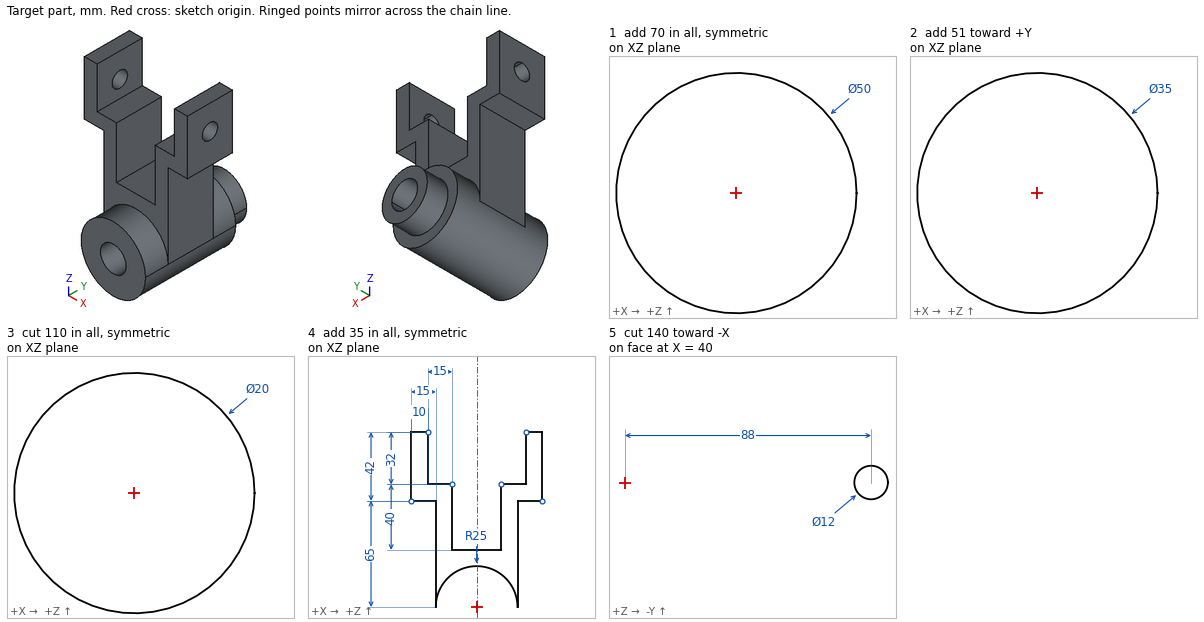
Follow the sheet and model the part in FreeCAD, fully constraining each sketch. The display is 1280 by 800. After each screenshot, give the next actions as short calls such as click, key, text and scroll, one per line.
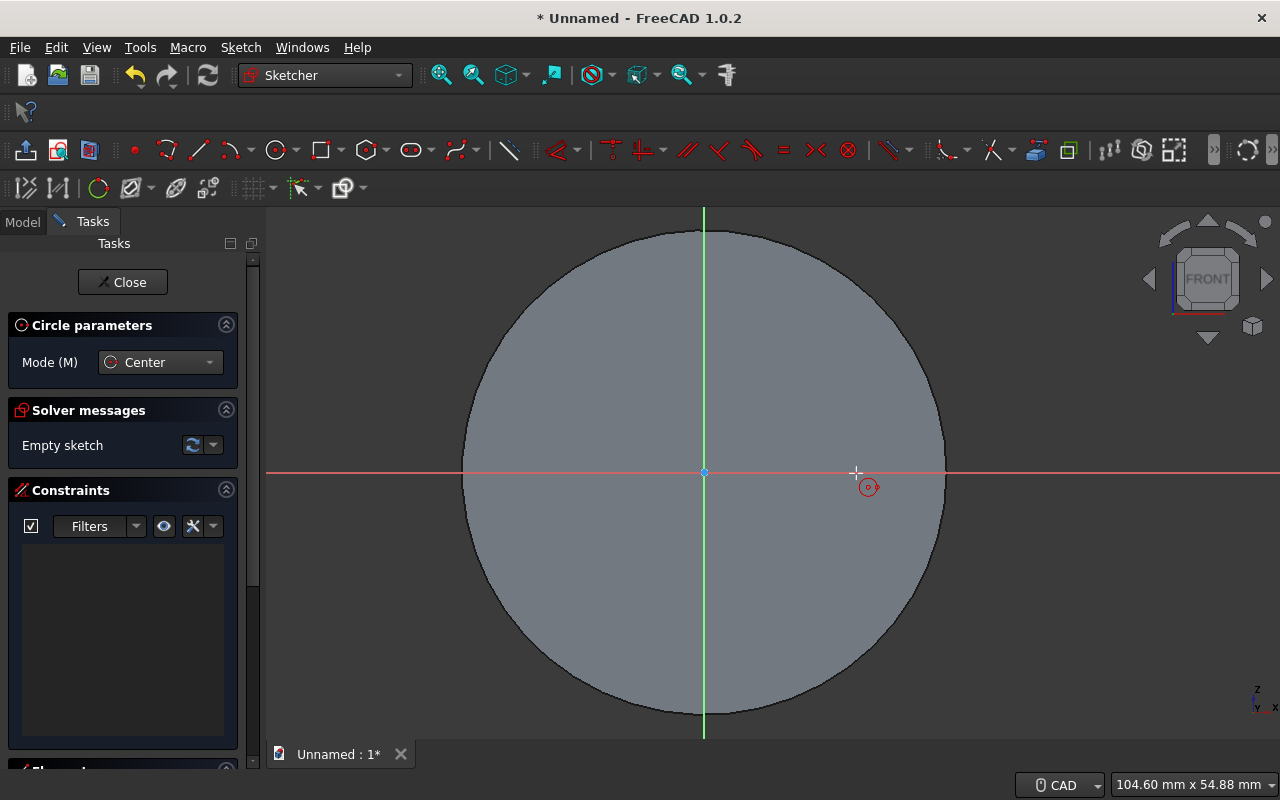
click(704, 473)
click(824, 353)
key(Escape)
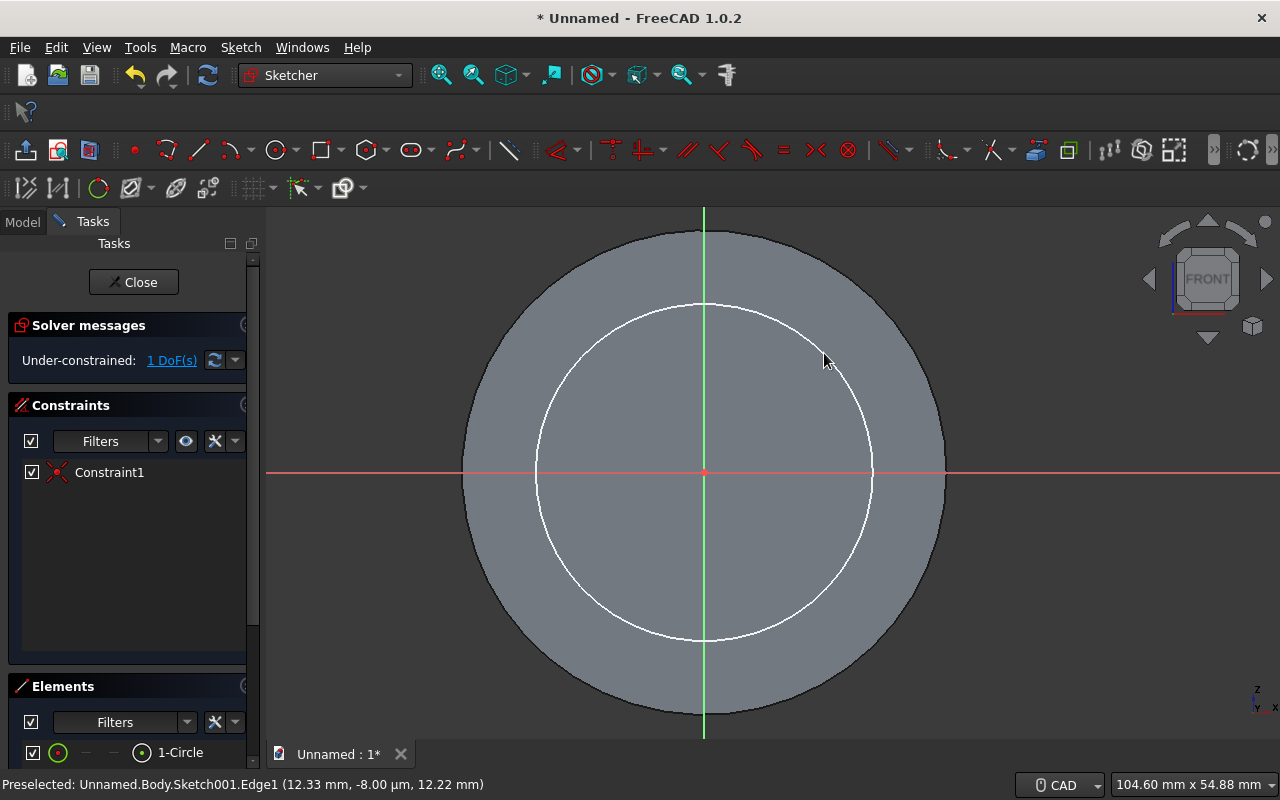
click(556, 150)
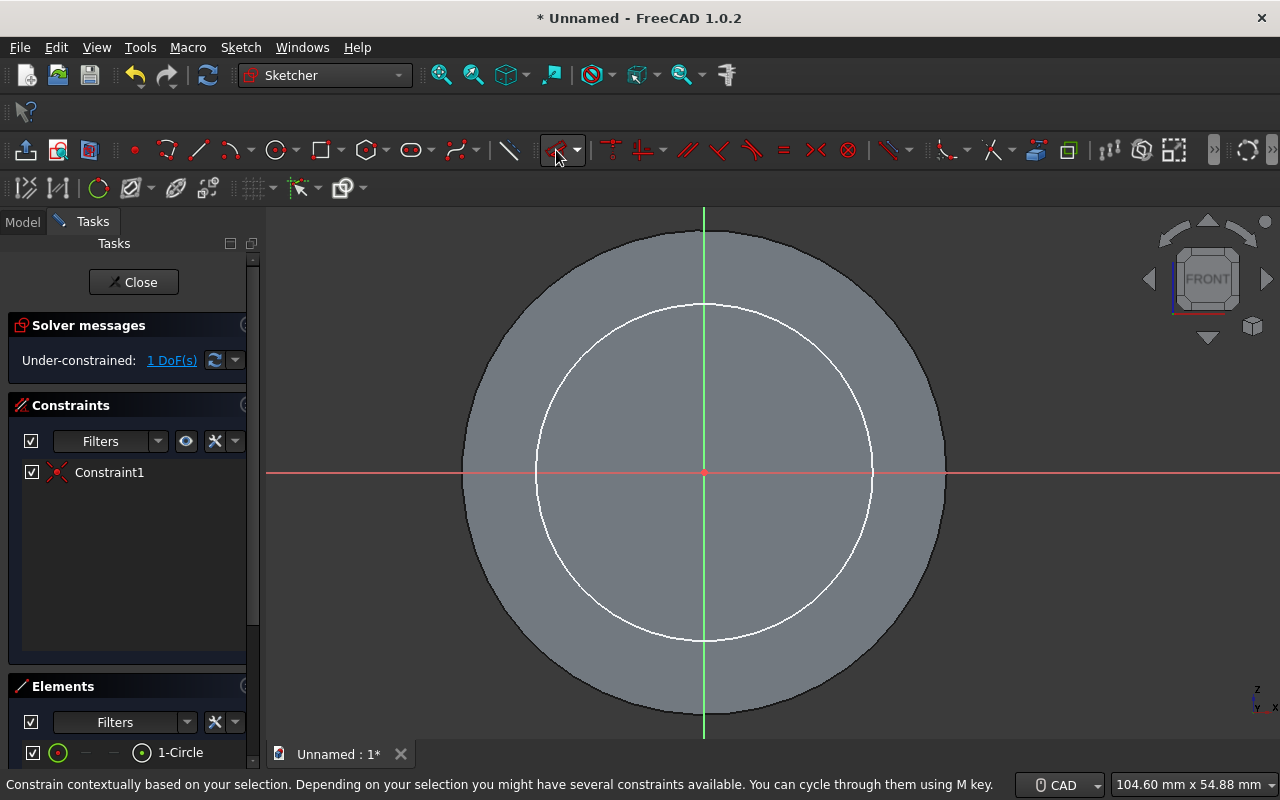
click(823, 353)
click(846, 330)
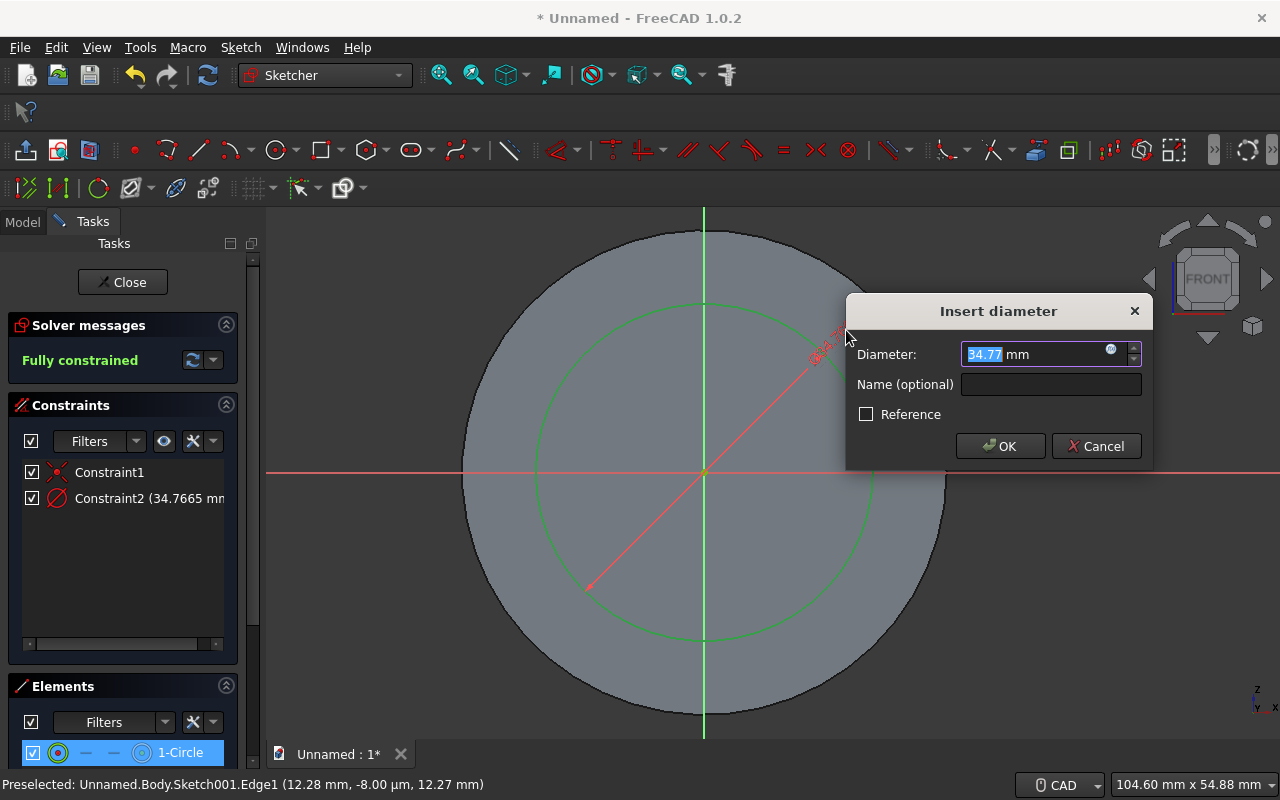
text(35)
key(Return)
key(Escape)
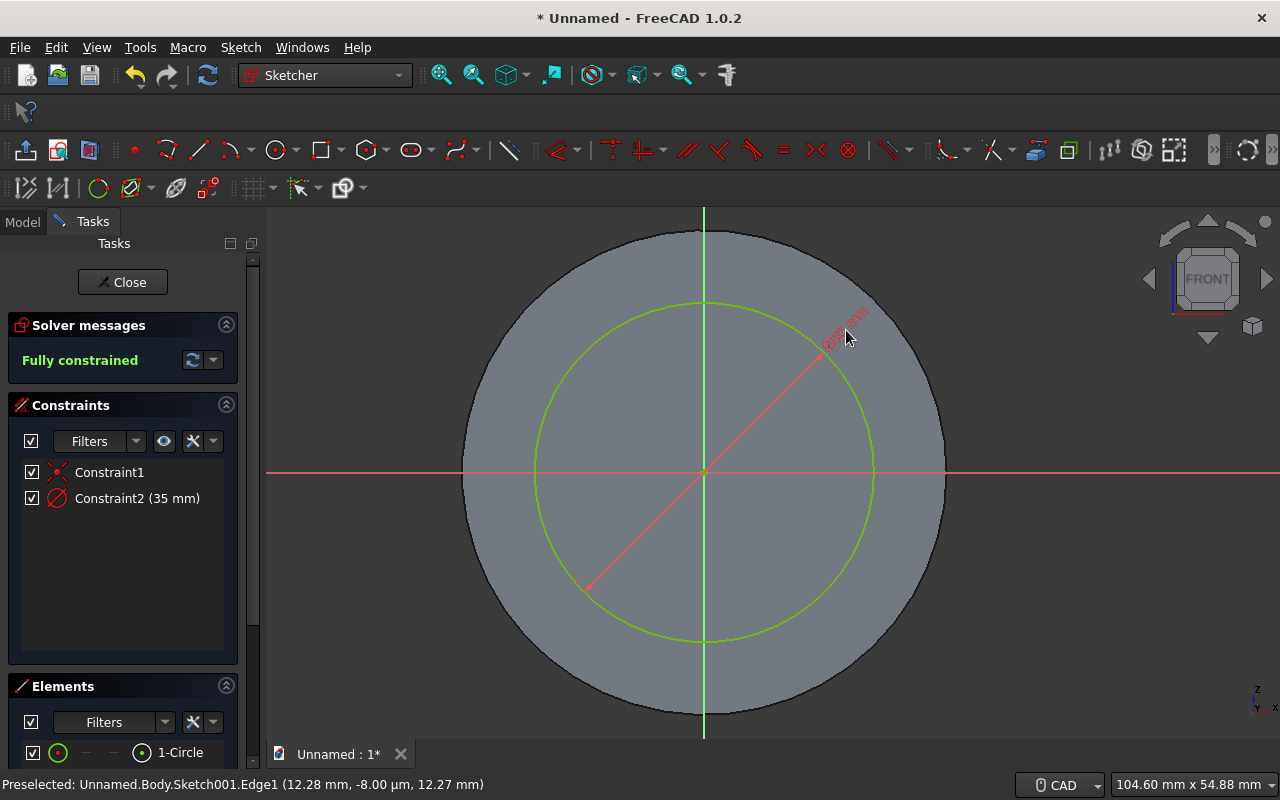
click(123, 282)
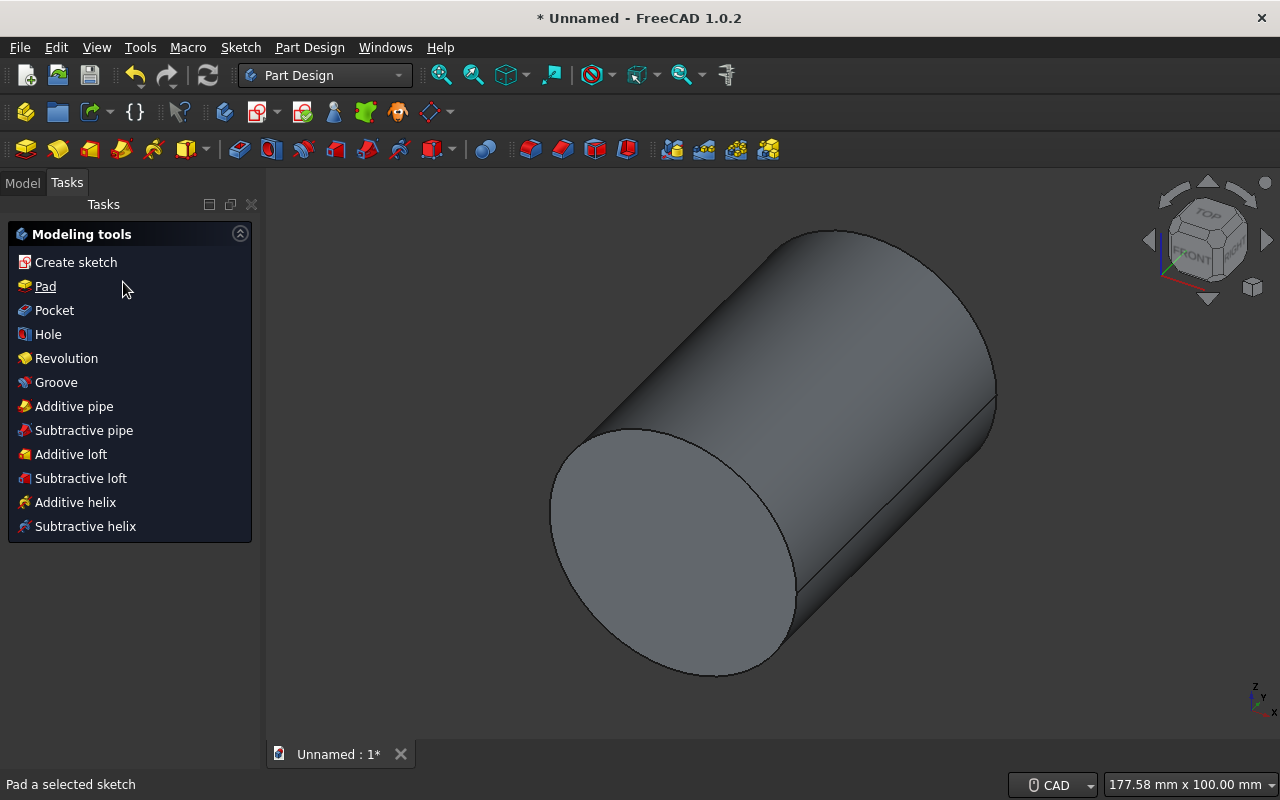
click(26, 150)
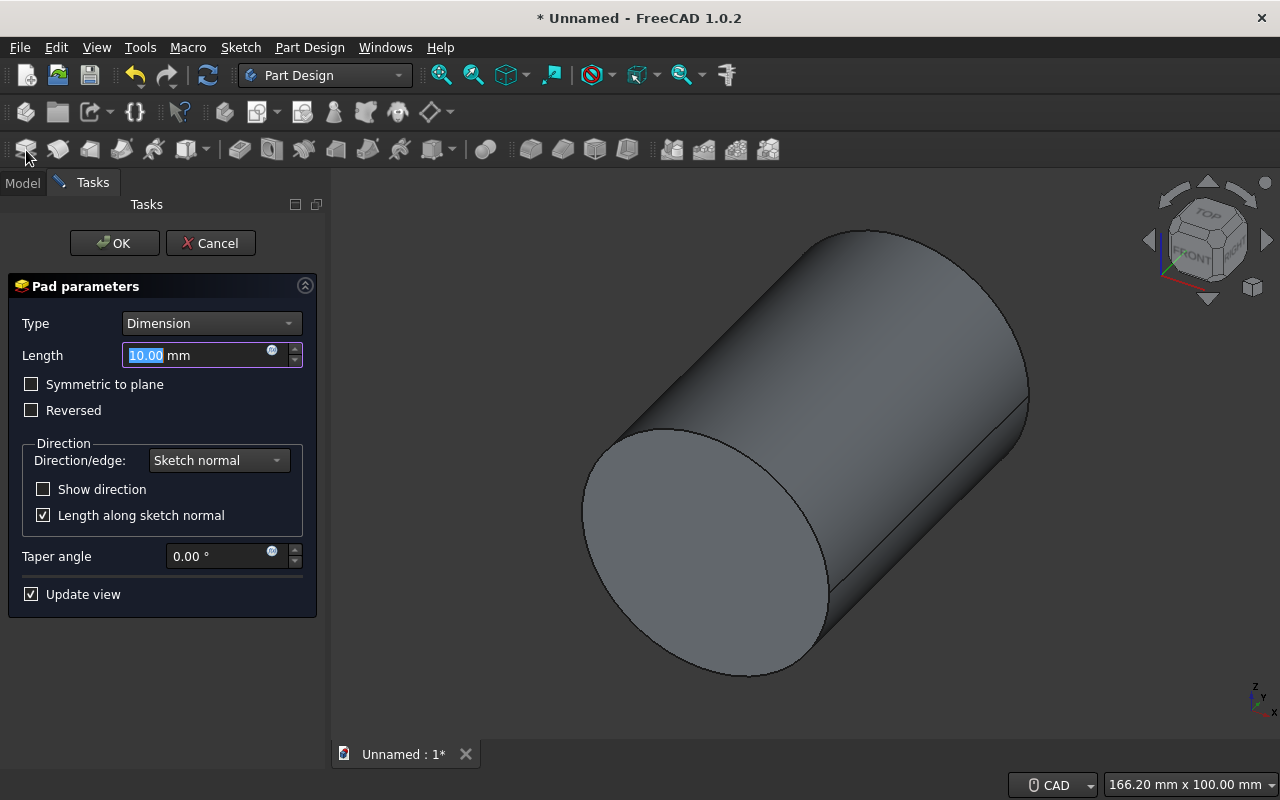
text(51)
key(Tab)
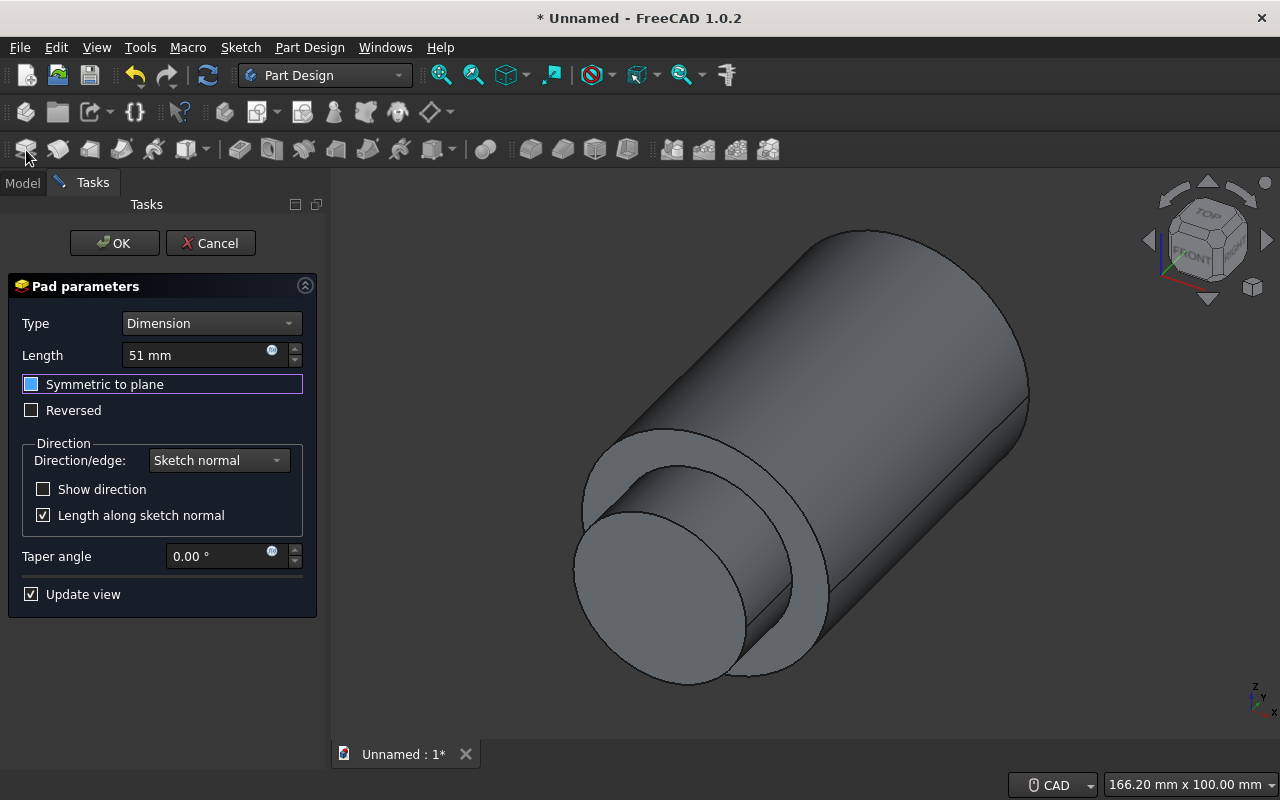
click(30, 410)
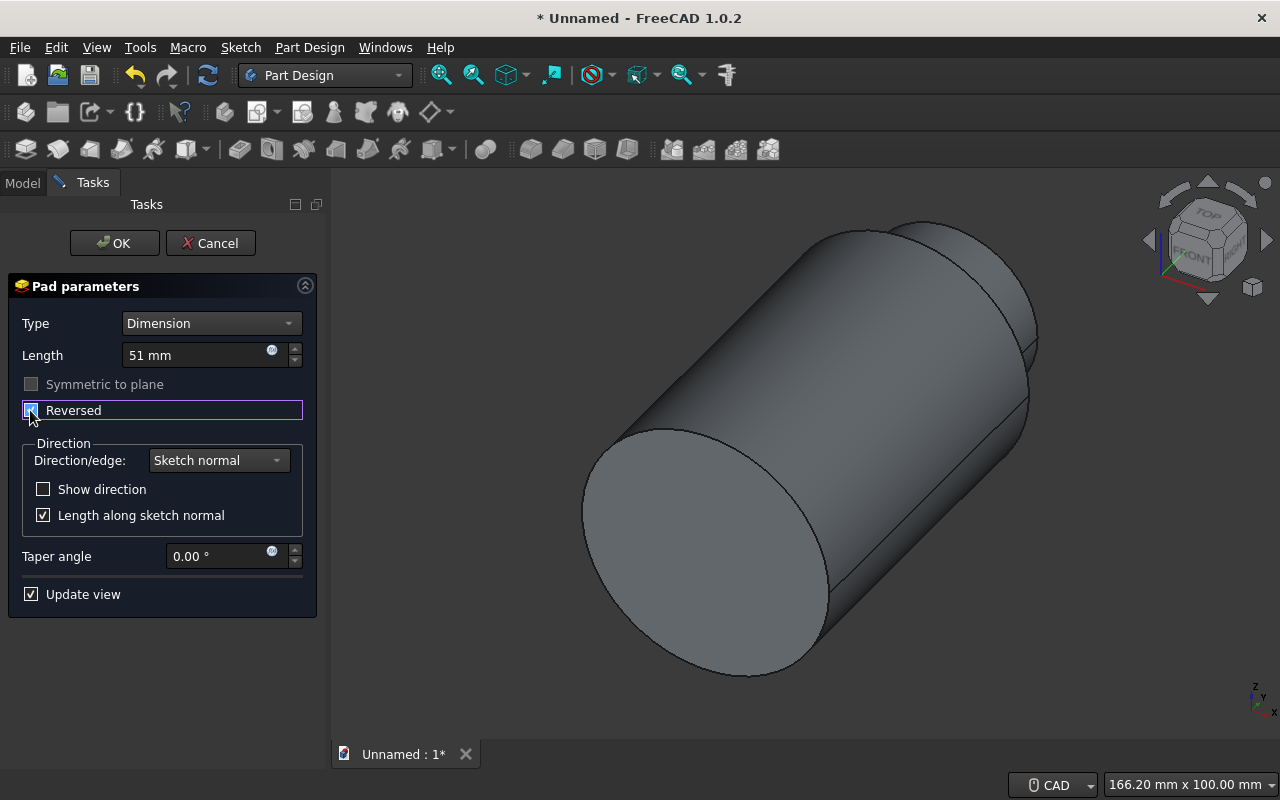
click(115, 243)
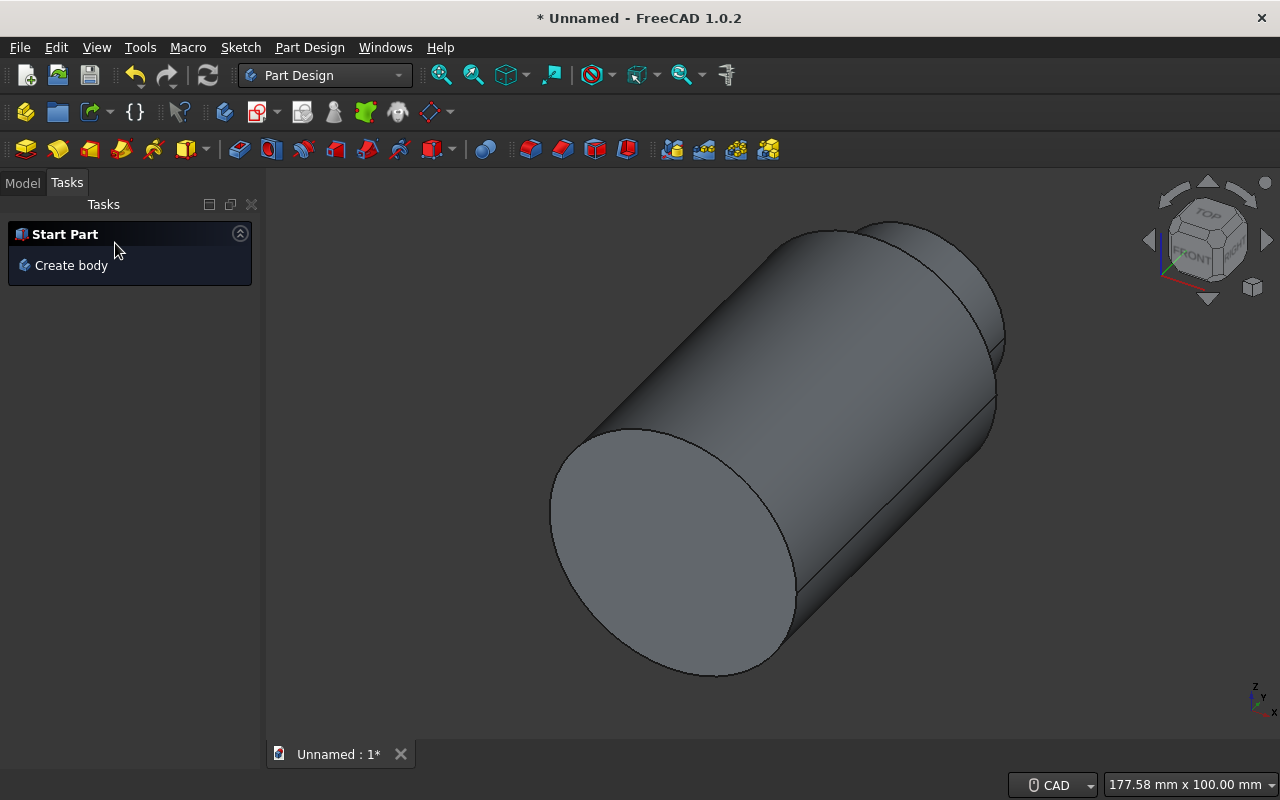
click(442, 76)